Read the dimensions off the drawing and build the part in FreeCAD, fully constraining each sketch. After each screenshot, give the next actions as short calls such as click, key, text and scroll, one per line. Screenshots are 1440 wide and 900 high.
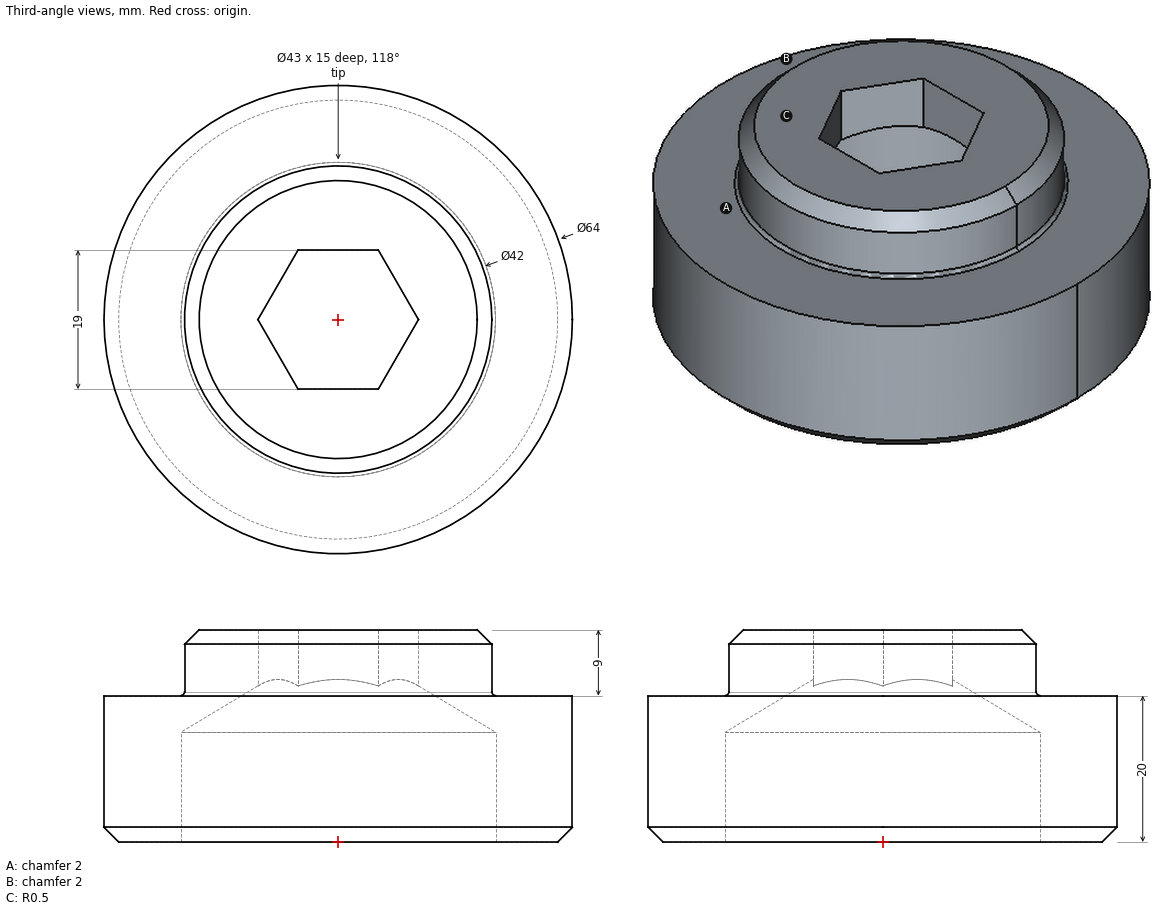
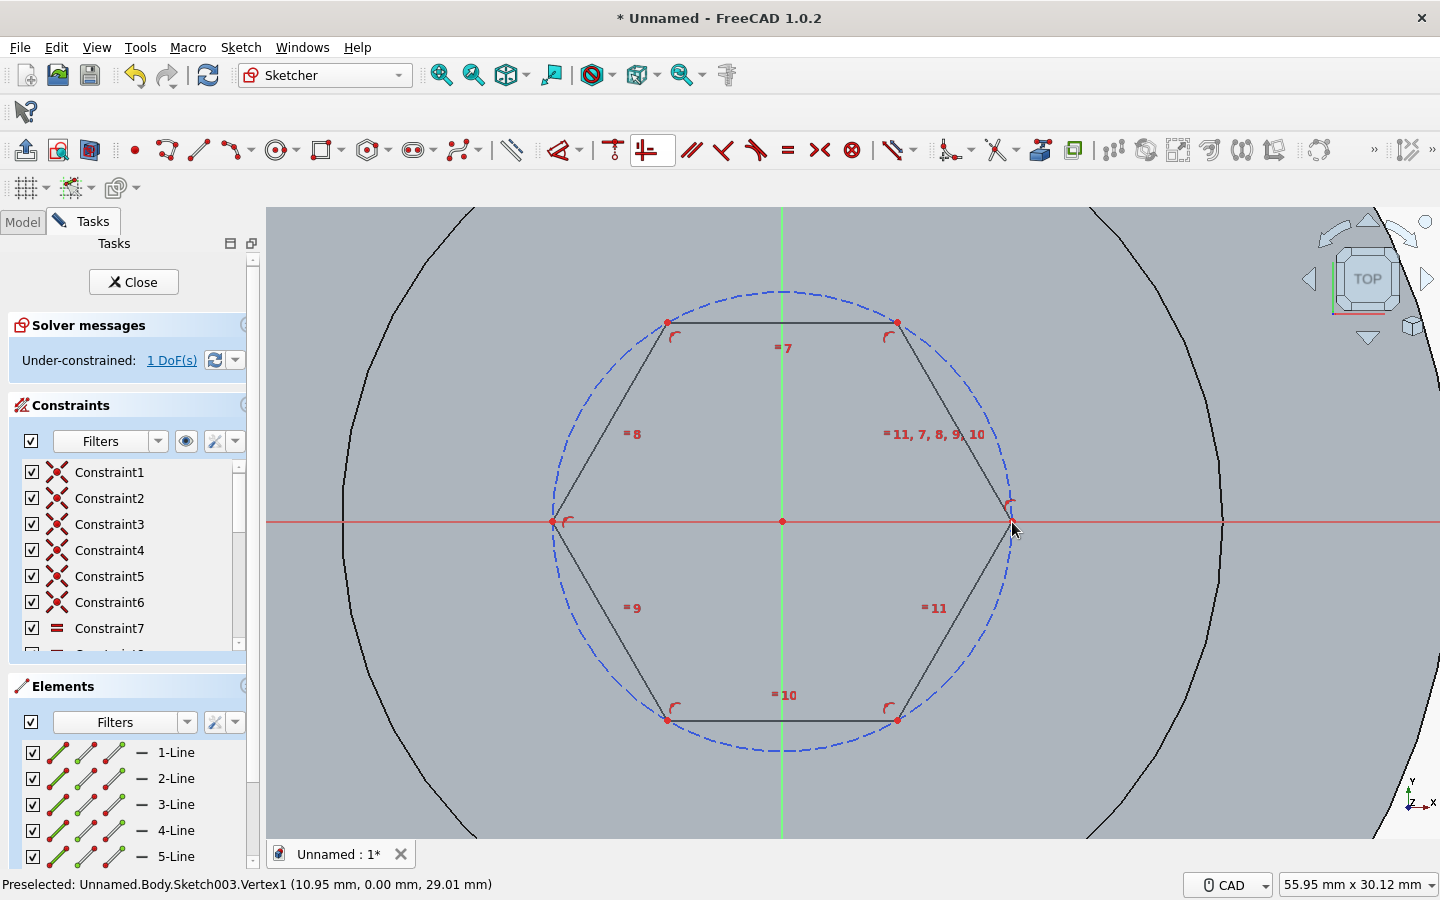
click(667, 721)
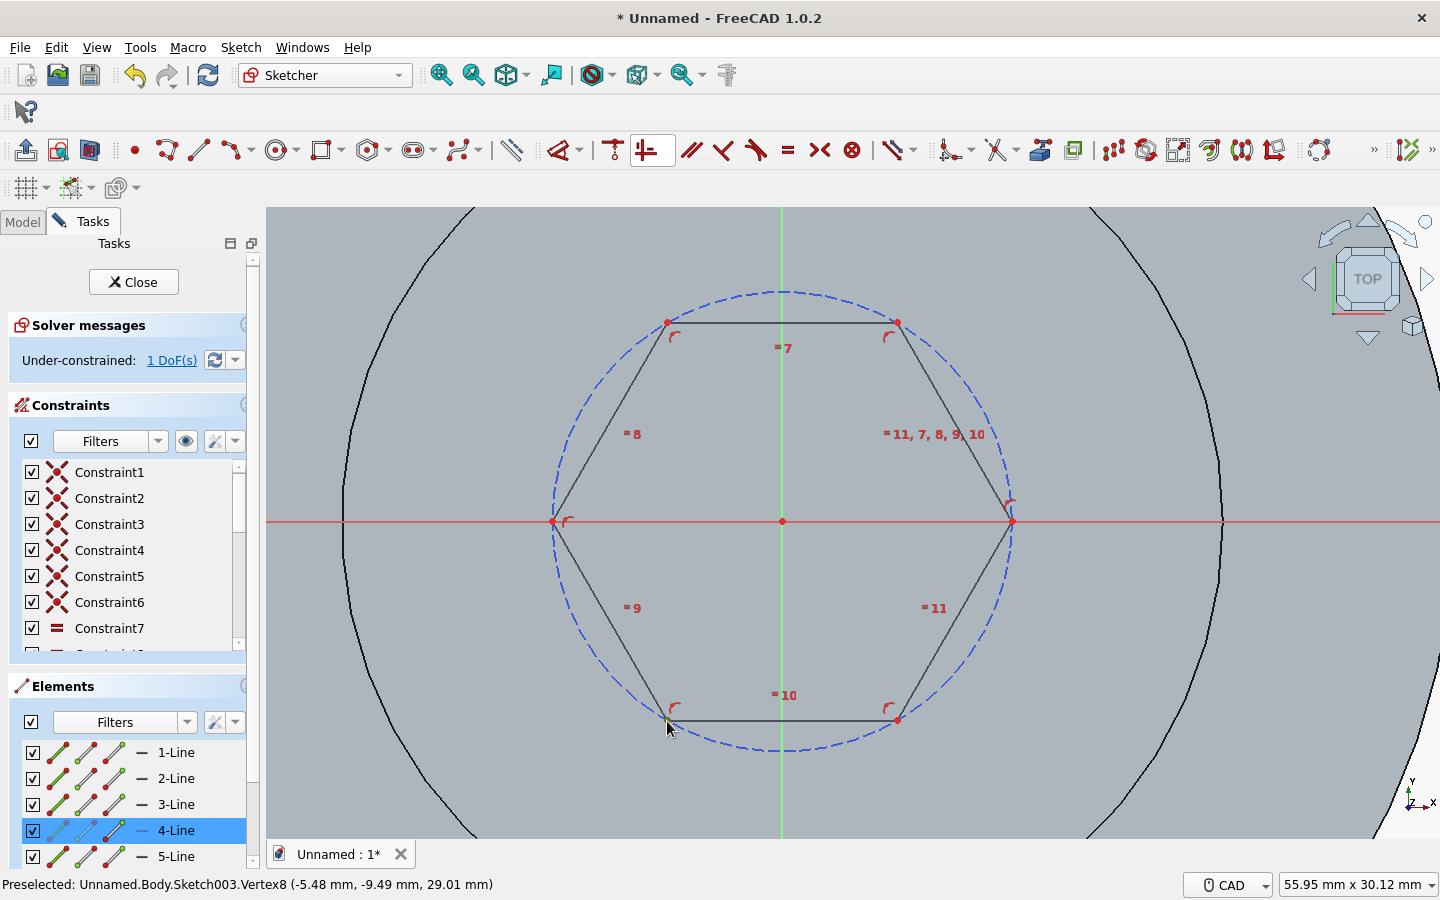
click(897, 323)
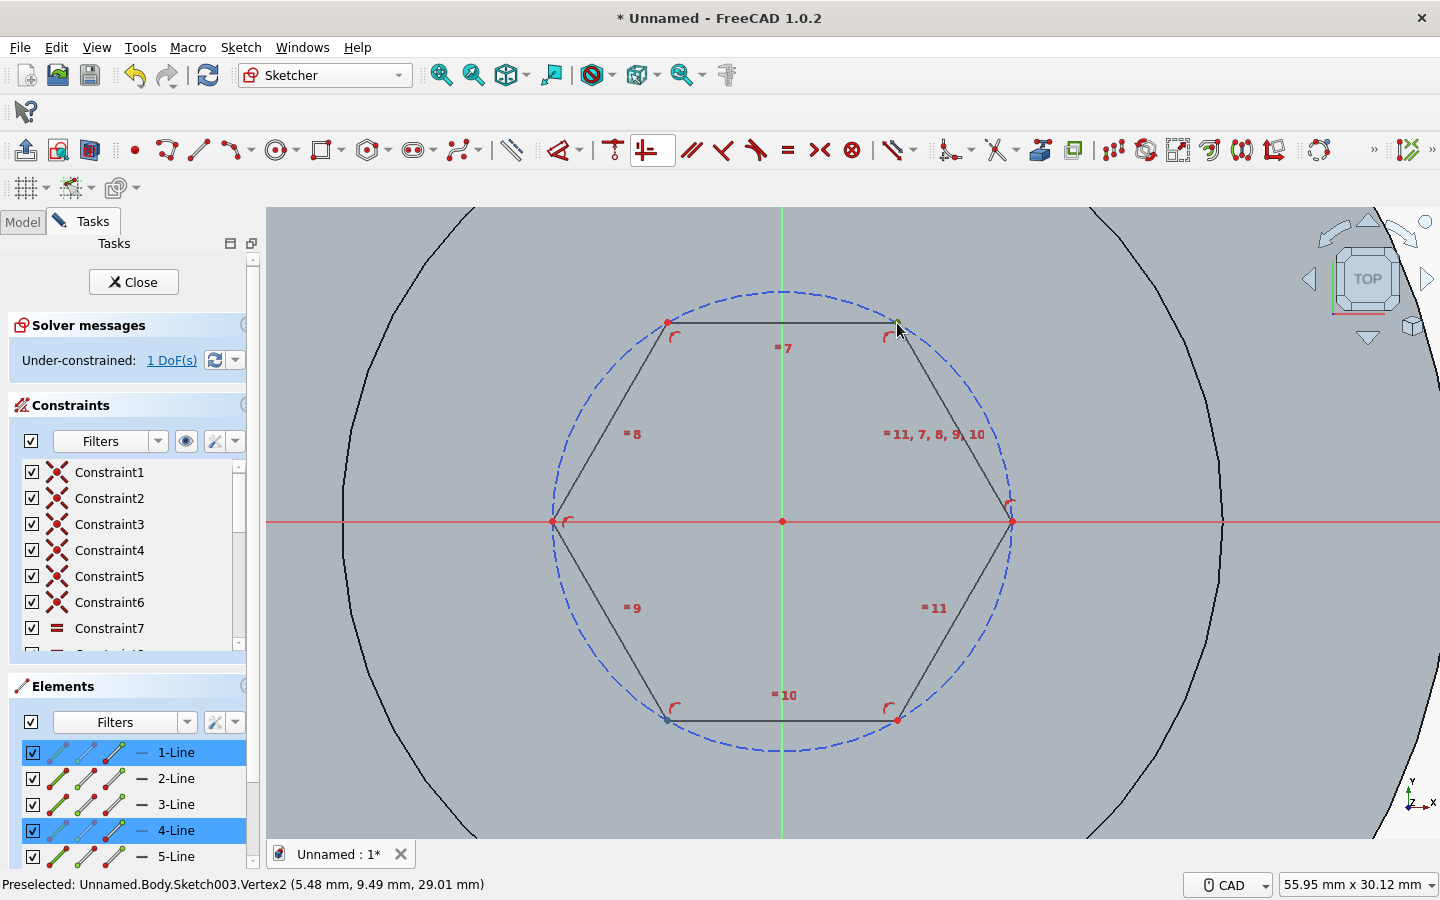
click(582, 150)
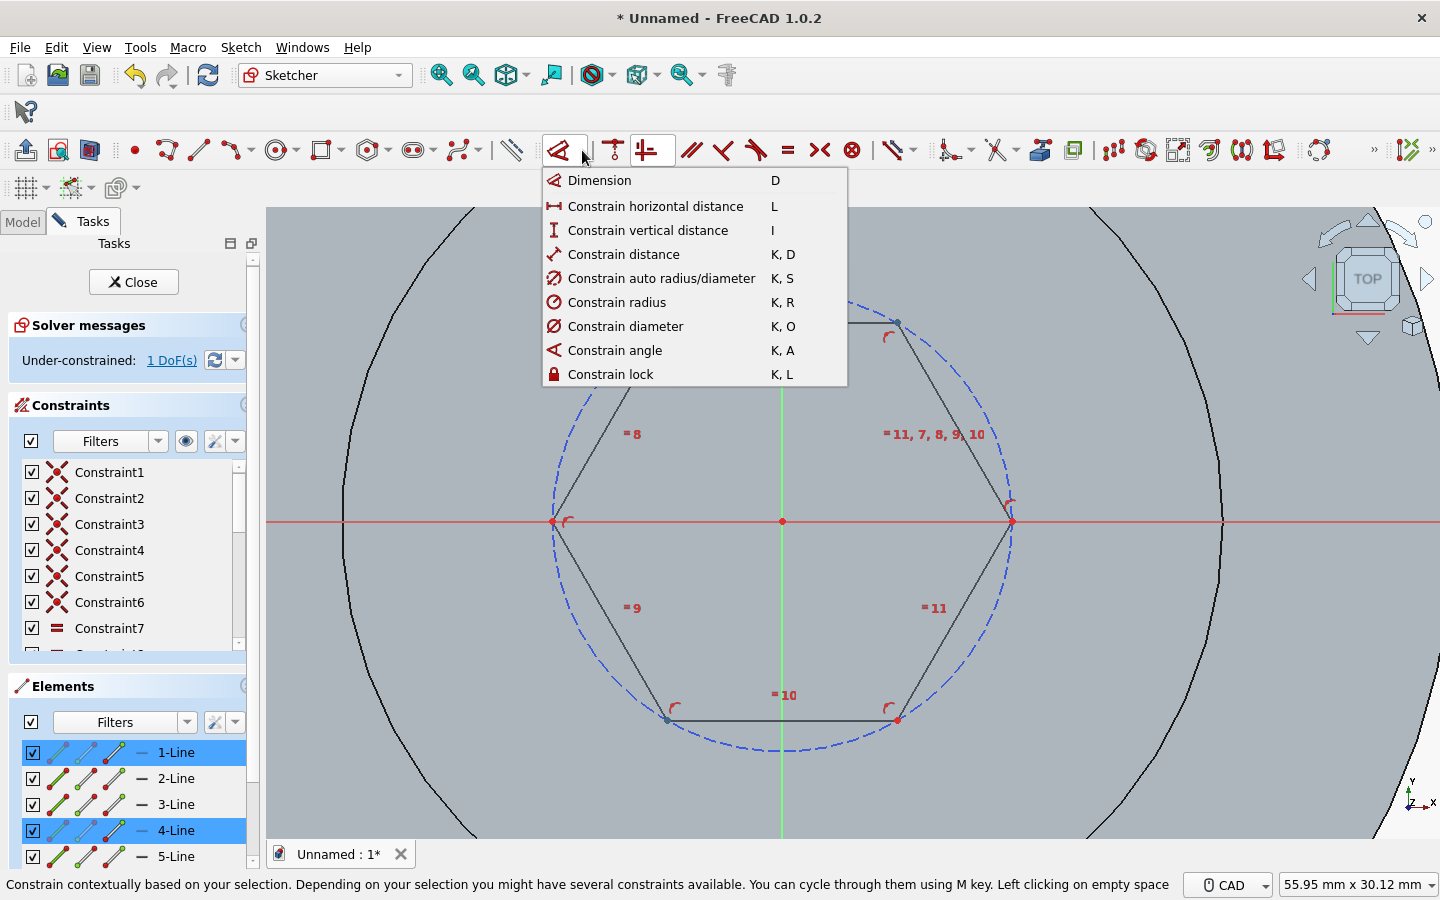
click(695, 230)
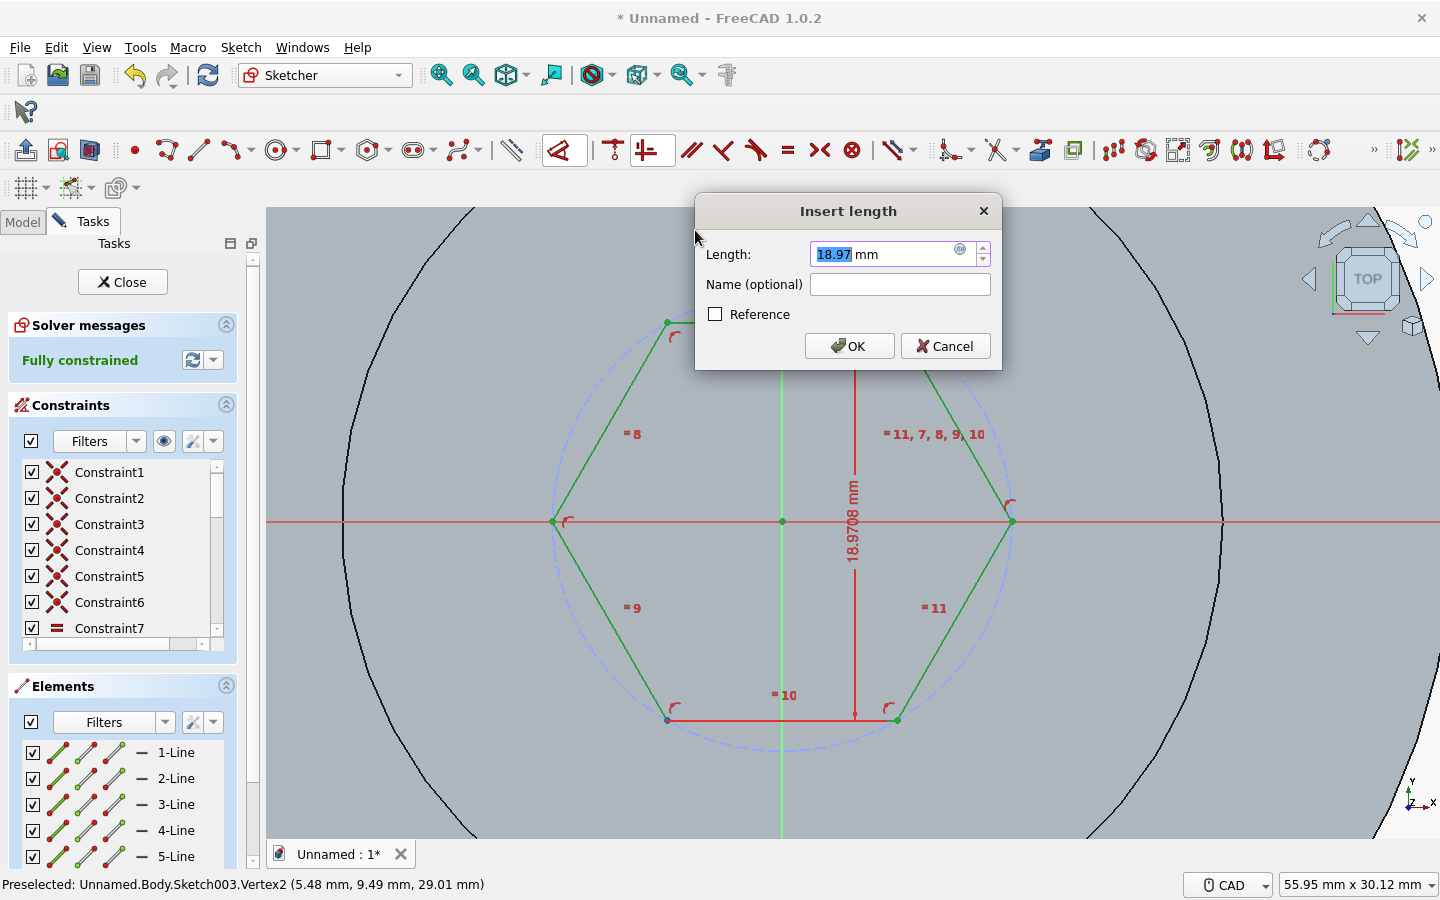
text(19)
key(Return)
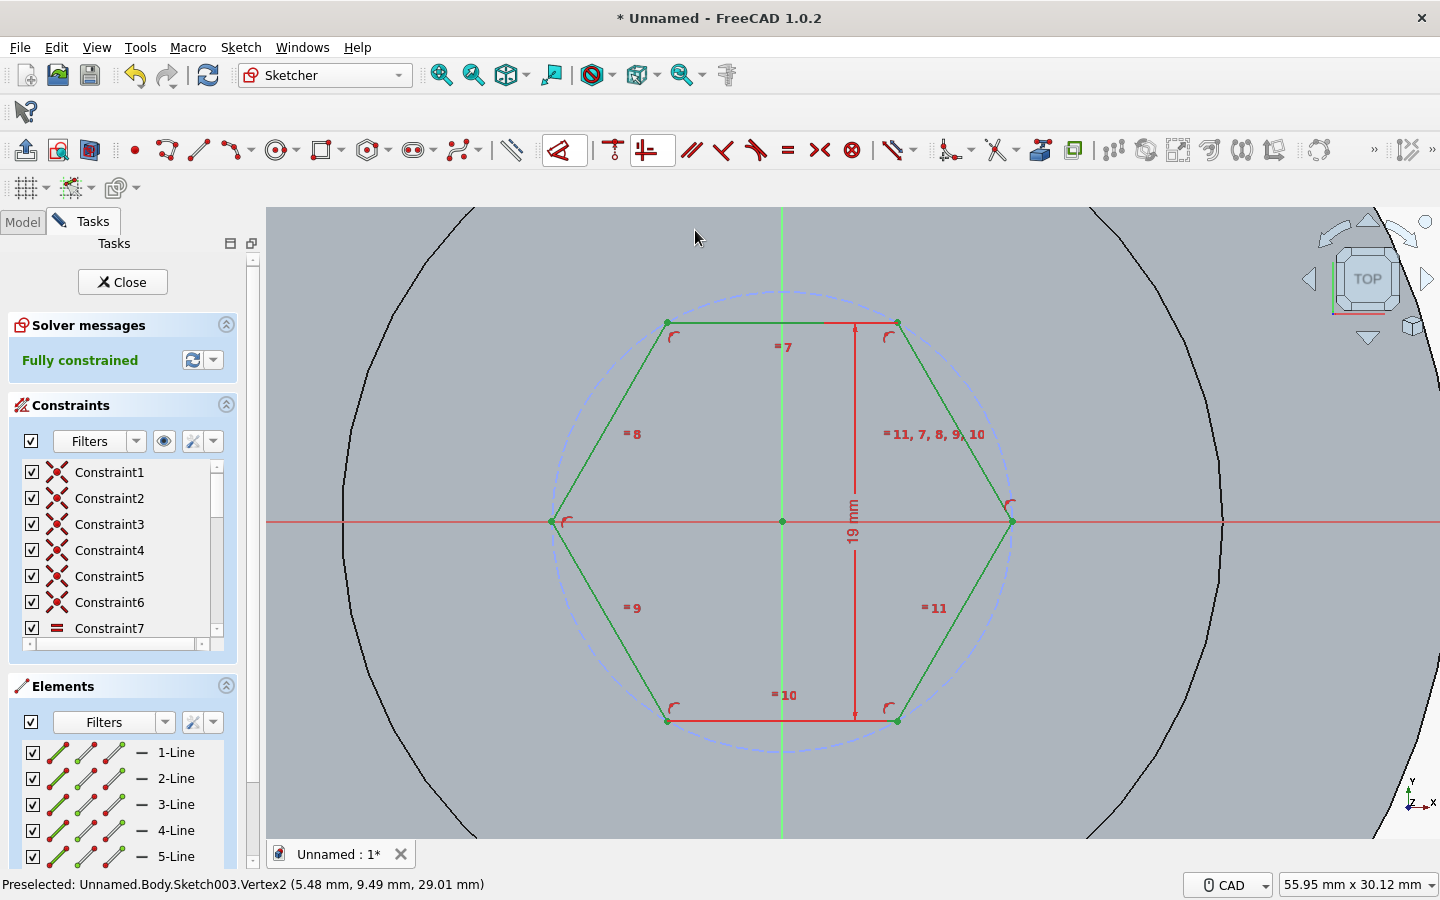
click(123, 282)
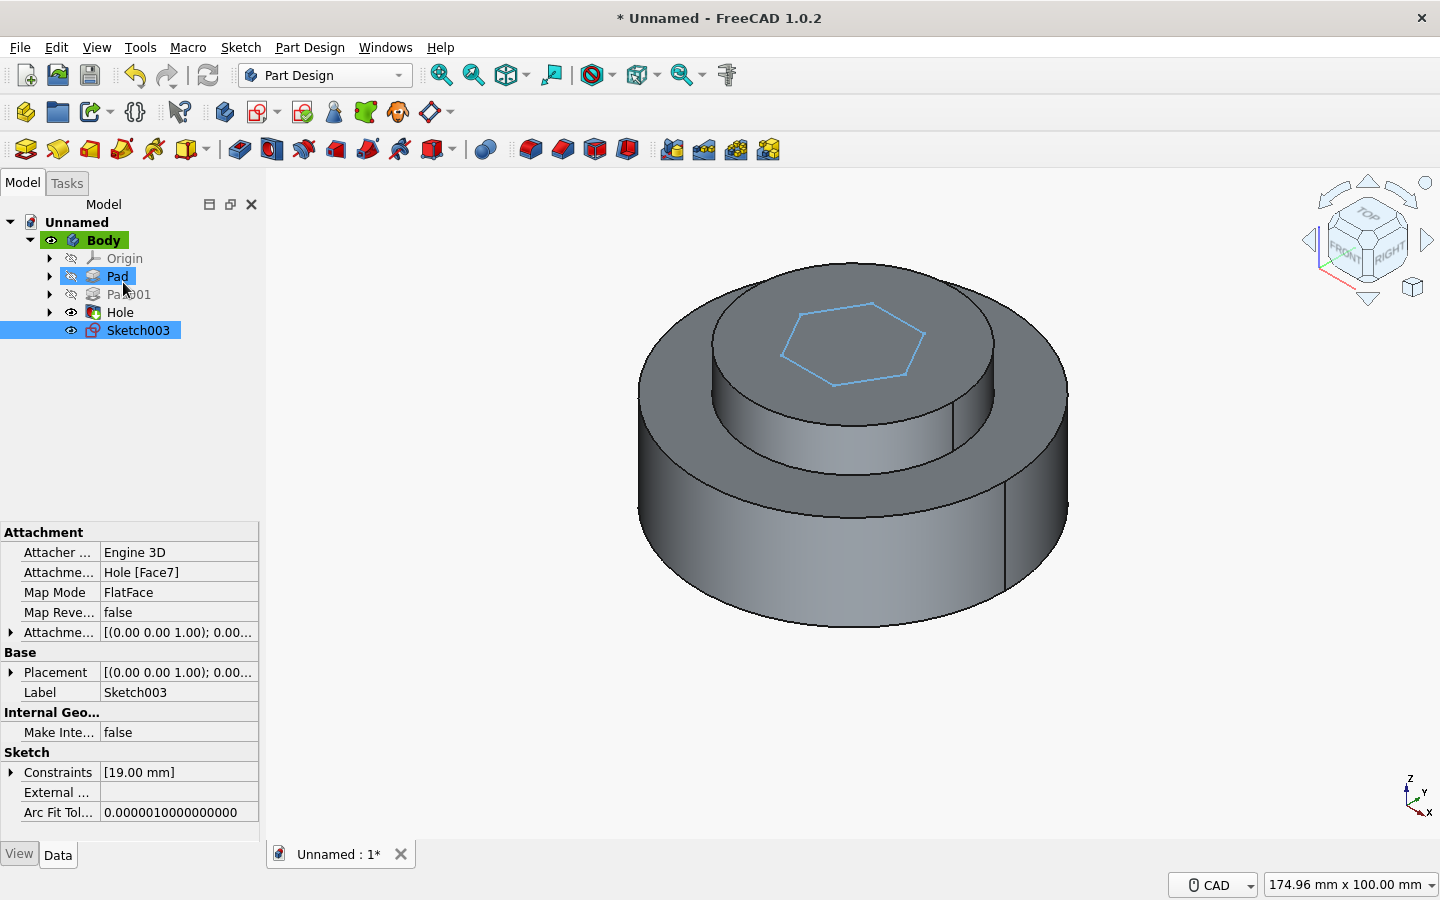
click(240, 150)